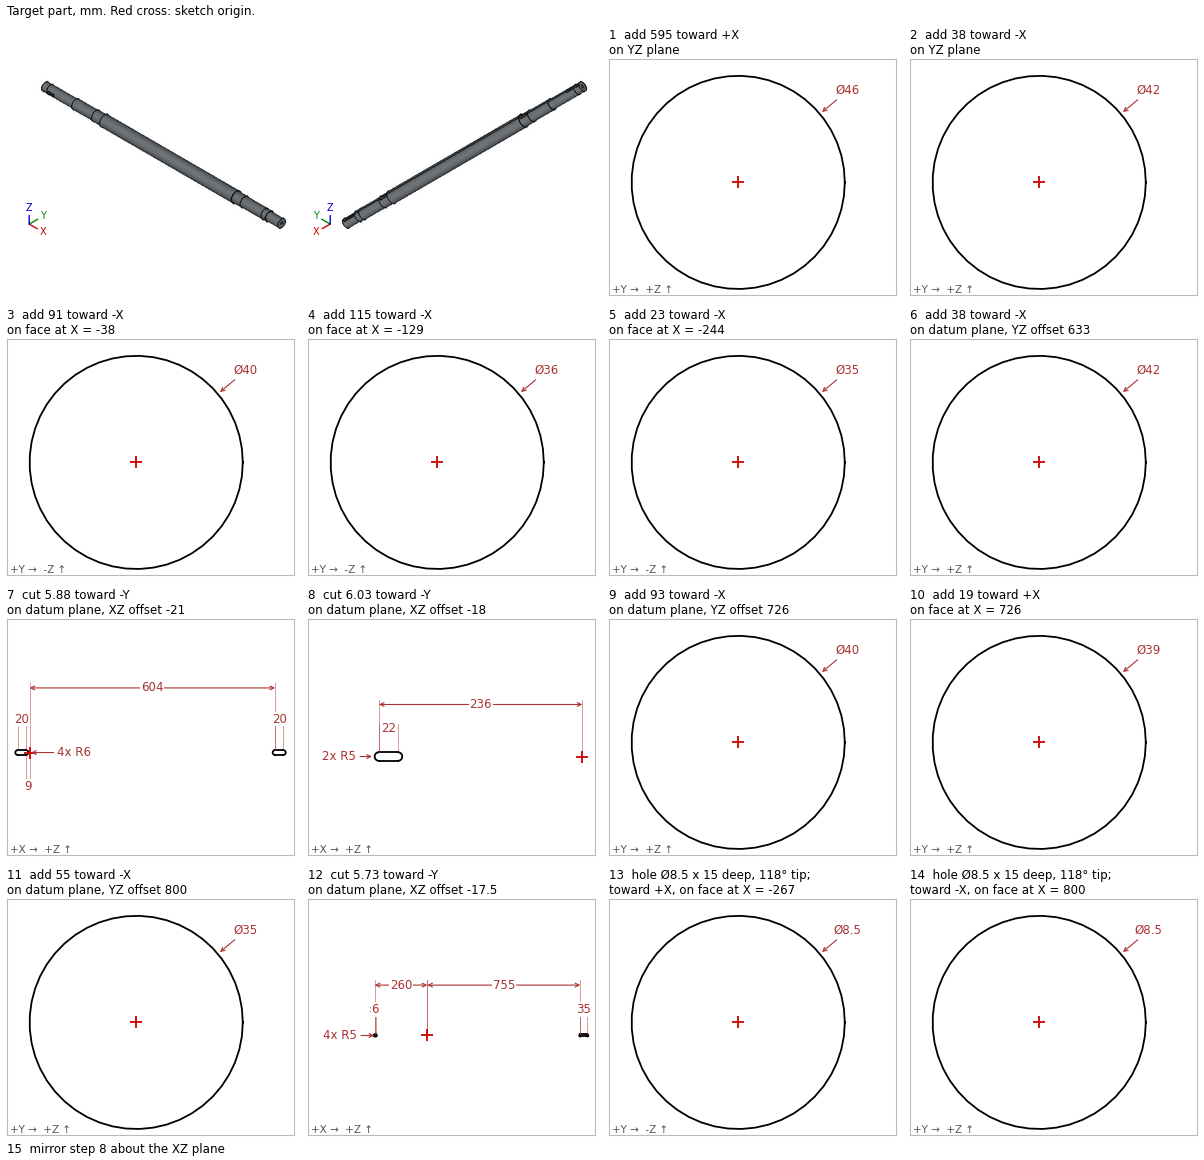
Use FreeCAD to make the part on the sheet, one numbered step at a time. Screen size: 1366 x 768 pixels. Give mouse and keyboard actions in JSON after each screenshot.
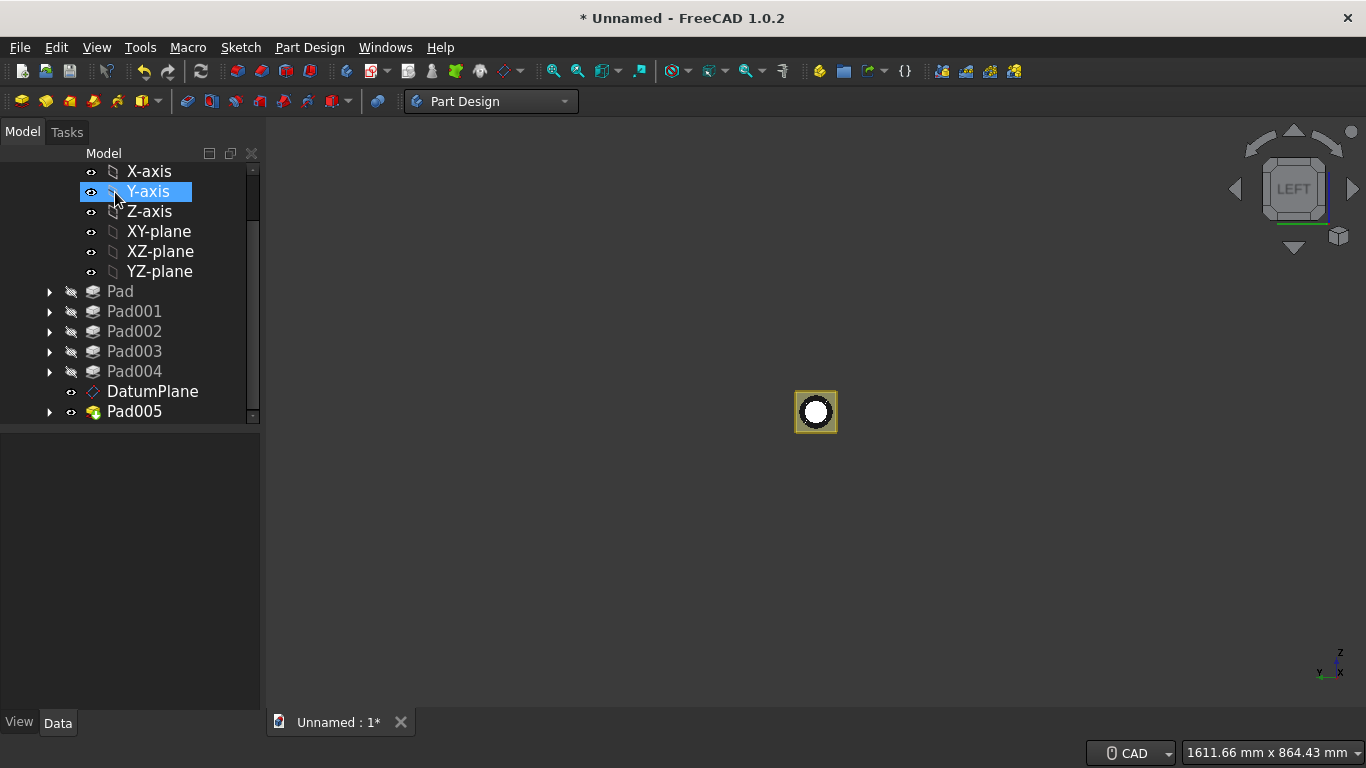
{"action": "left_click", "coordinate": [116, 392]}
{"action": "key", "text": "space"}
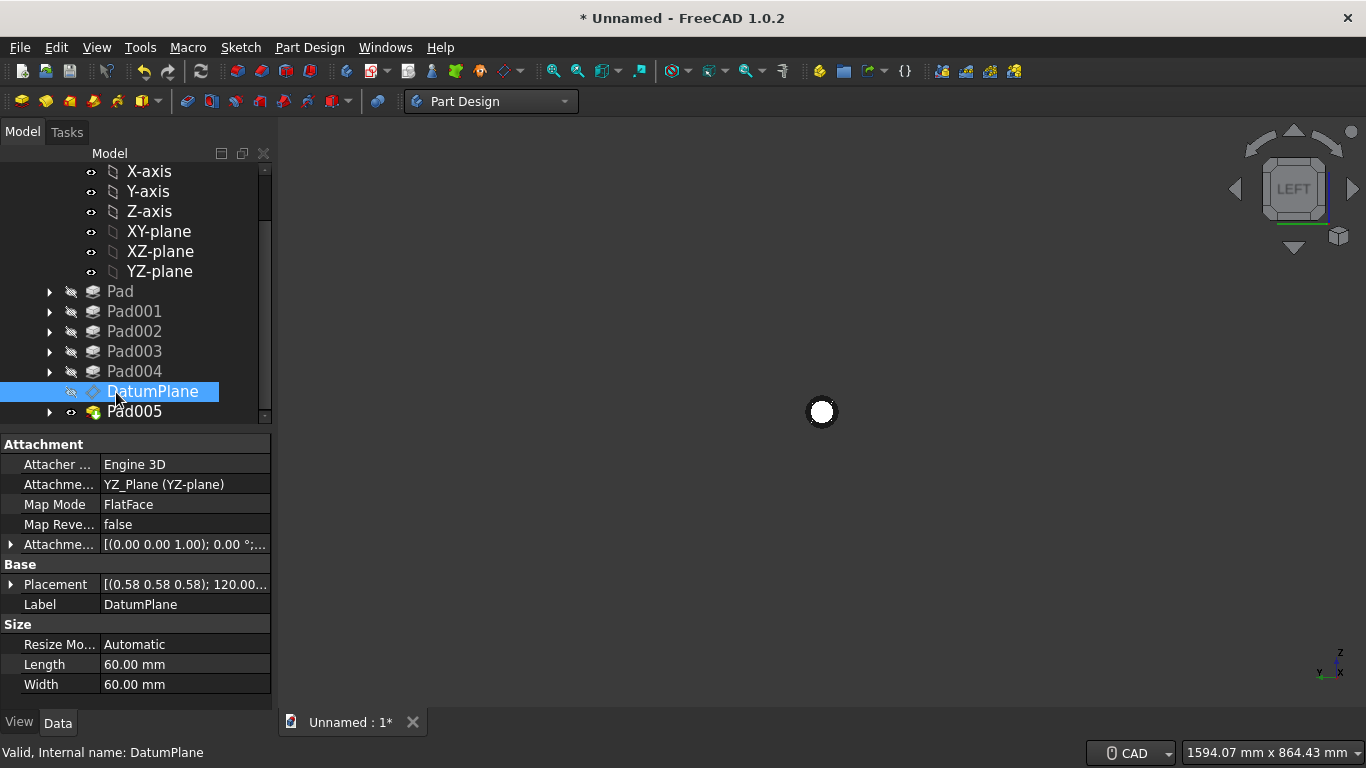
{"action": "key", "text": "v f"}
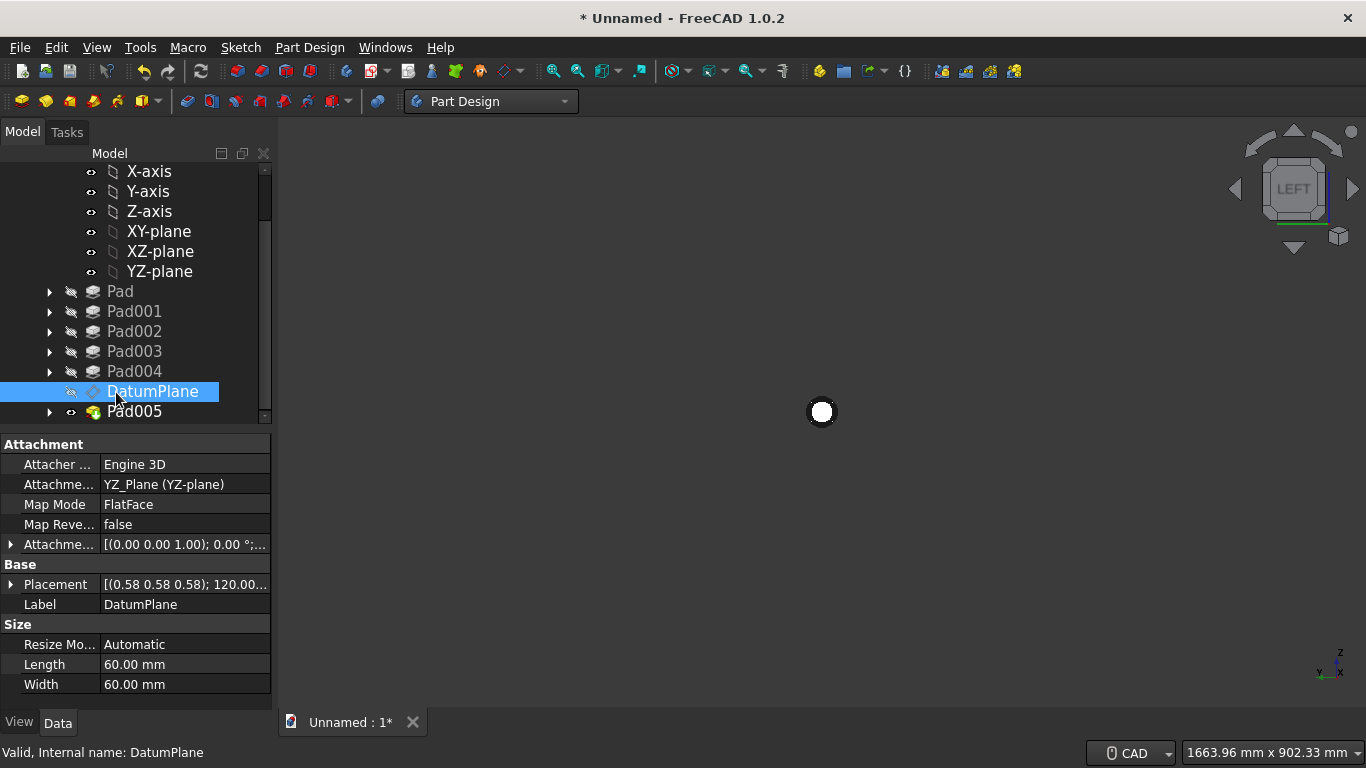
{"action": "scroll", "coordinate": [160, 287], "scroll_direction": "down", "scroll_amount": 3}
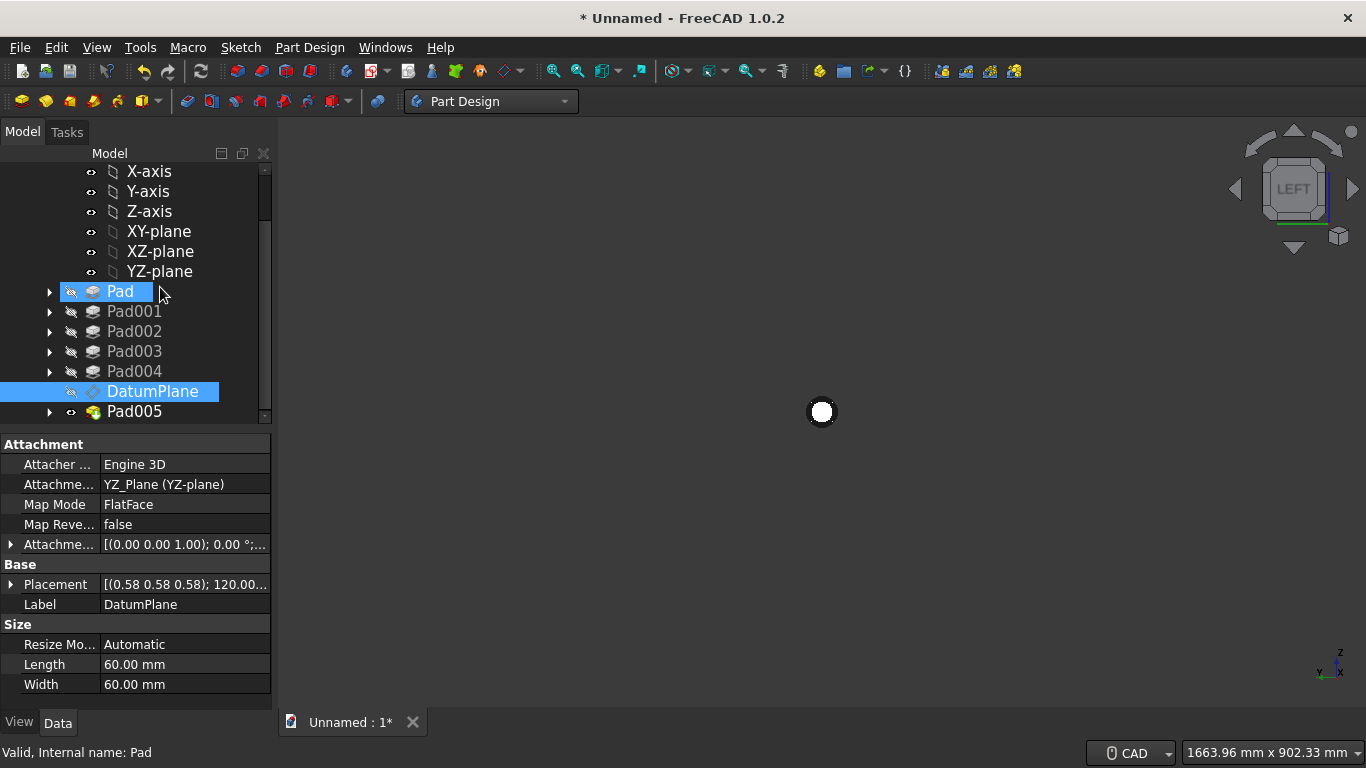
{"action": "scroll", "coordinate": [160, 287], "scroll_direction": "up", "scroll_amount": 15}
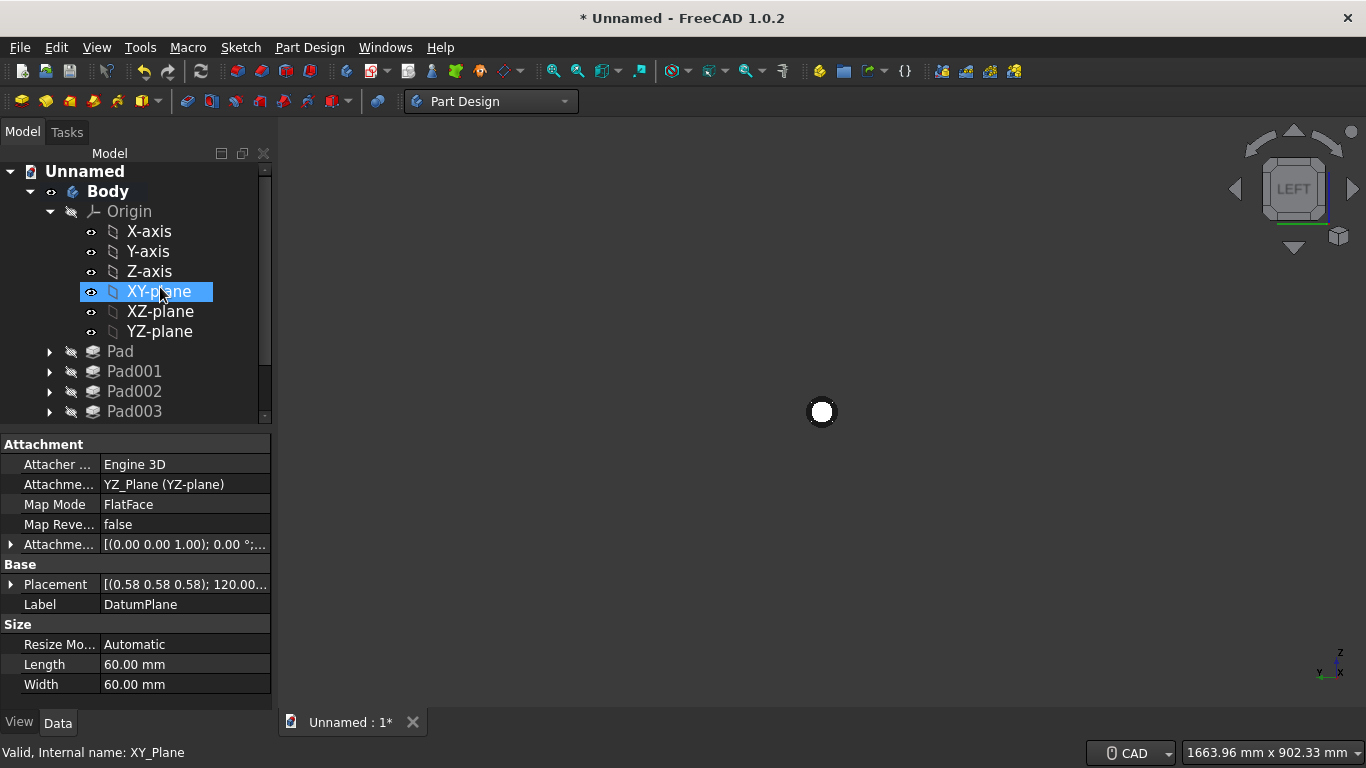
{"action": "left_click", "coordinate": [136, 312]}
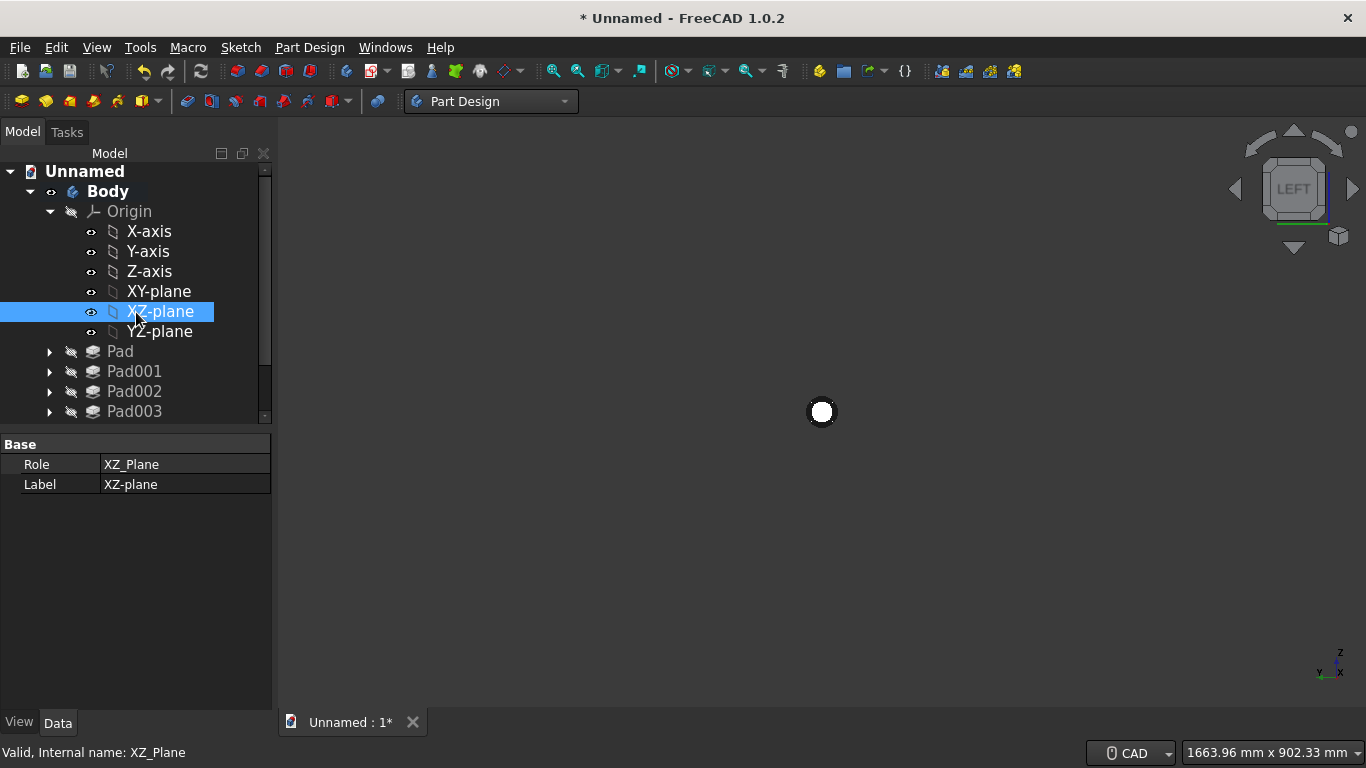
{"action": "left_click", "coordinate": [504, 72]}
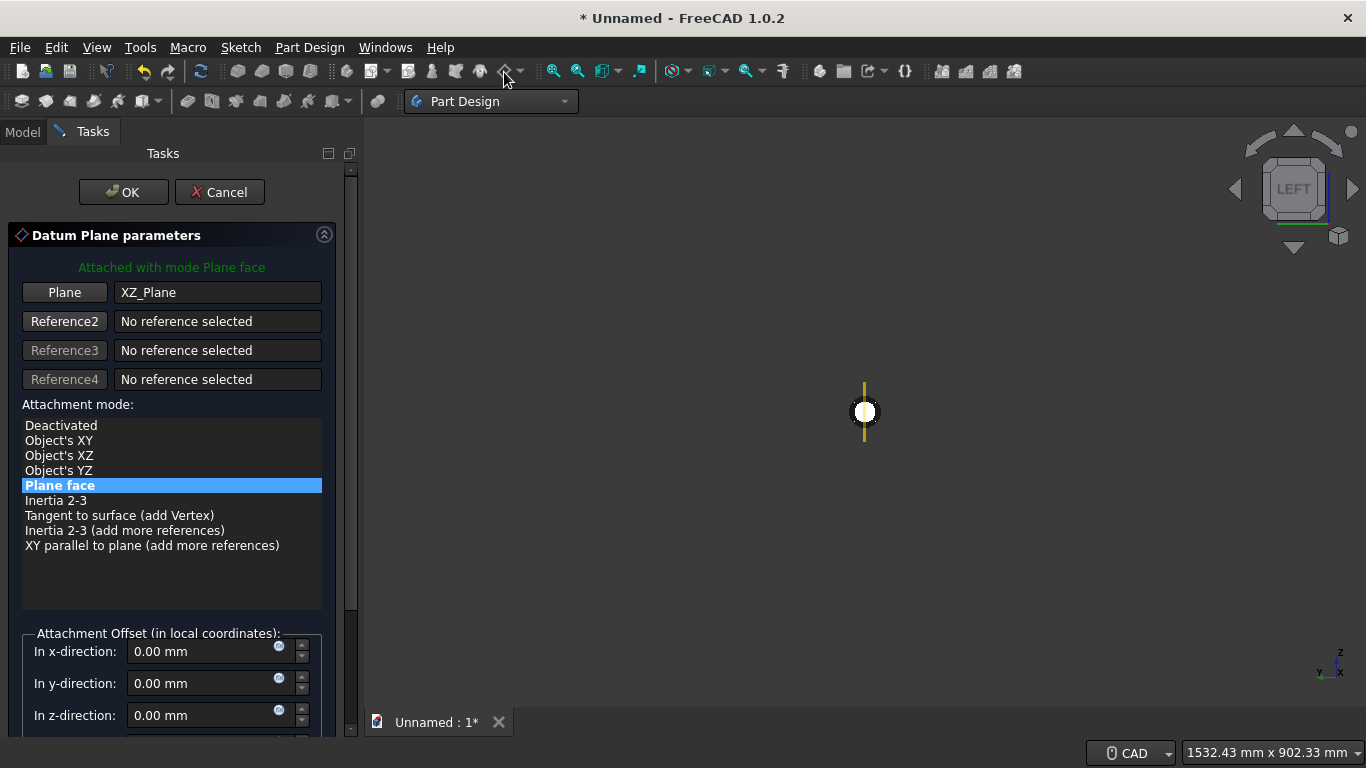
{"action": "triple_click", "coordinate": [210, 715]}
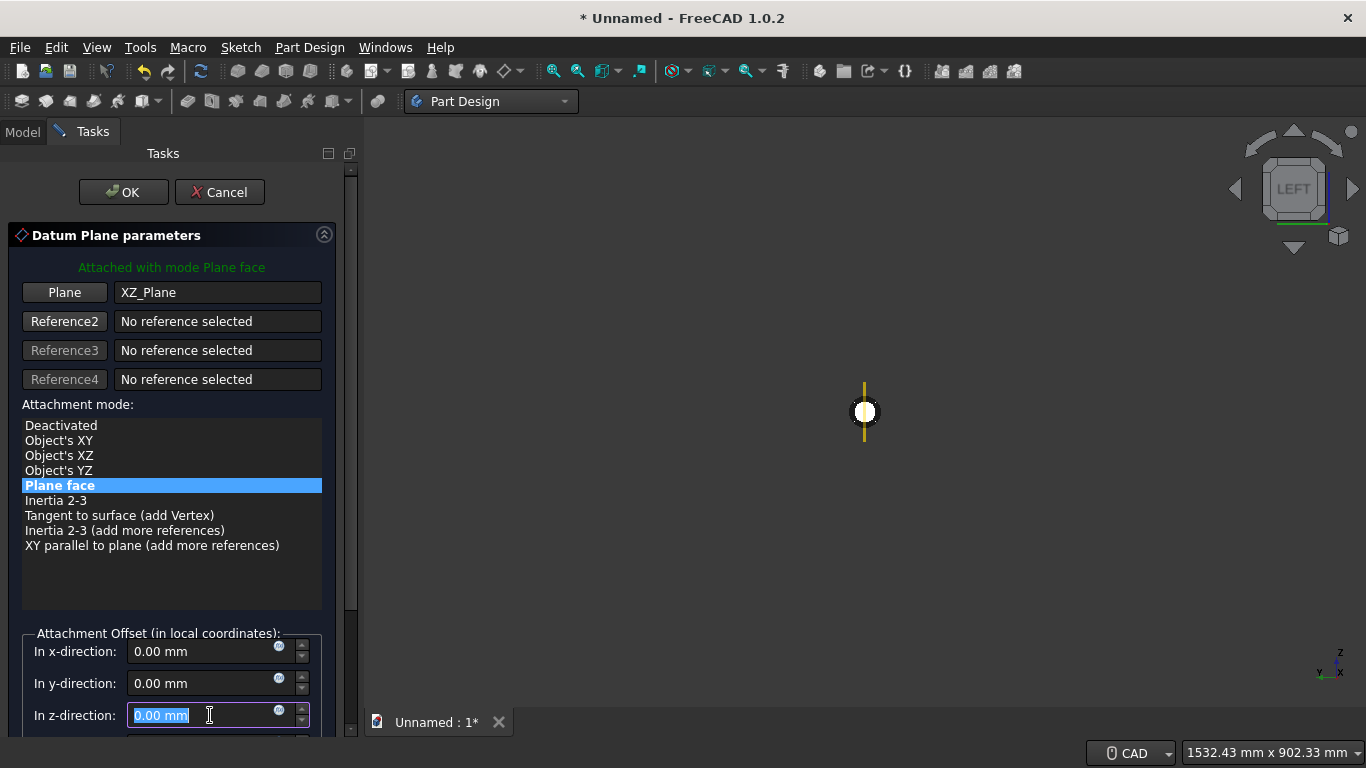
{"action": "type", "text": "-21"}
{"action": "key", "text": "Tab"}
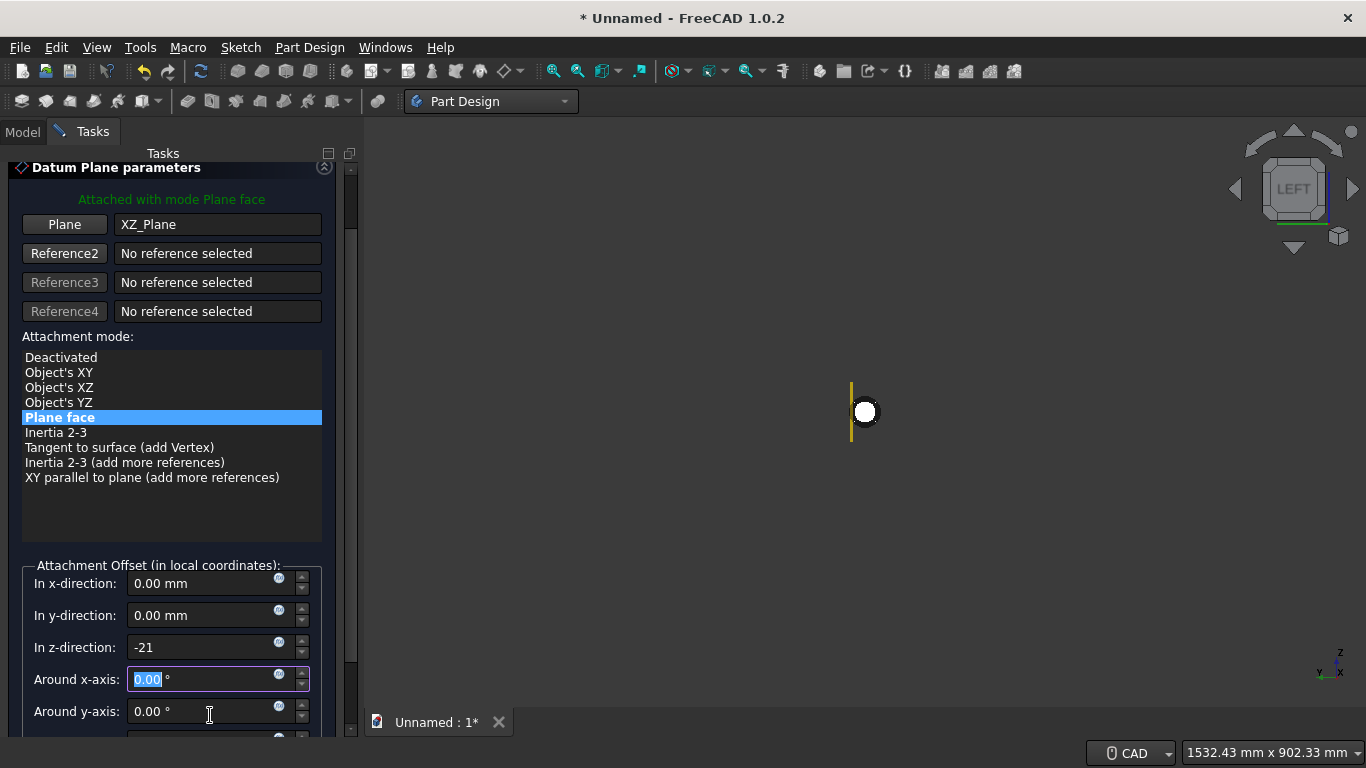
{"action": "scroll", "coordinate": [351, 450], "scroll_direction": "up", "scroll_amount": 2}